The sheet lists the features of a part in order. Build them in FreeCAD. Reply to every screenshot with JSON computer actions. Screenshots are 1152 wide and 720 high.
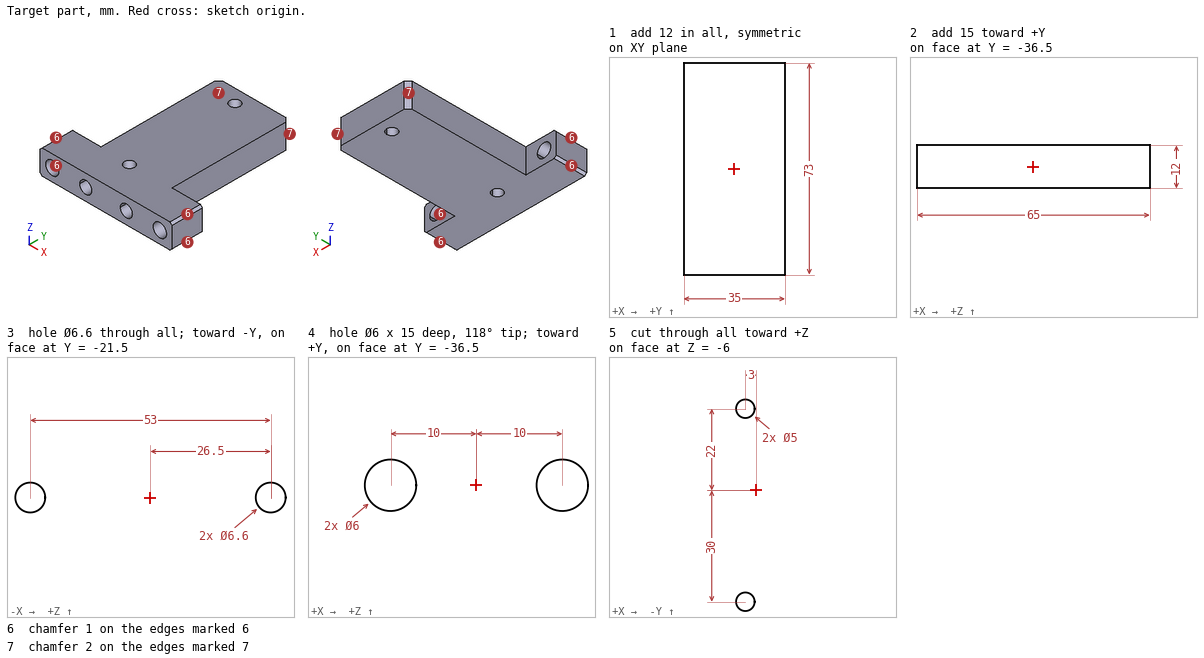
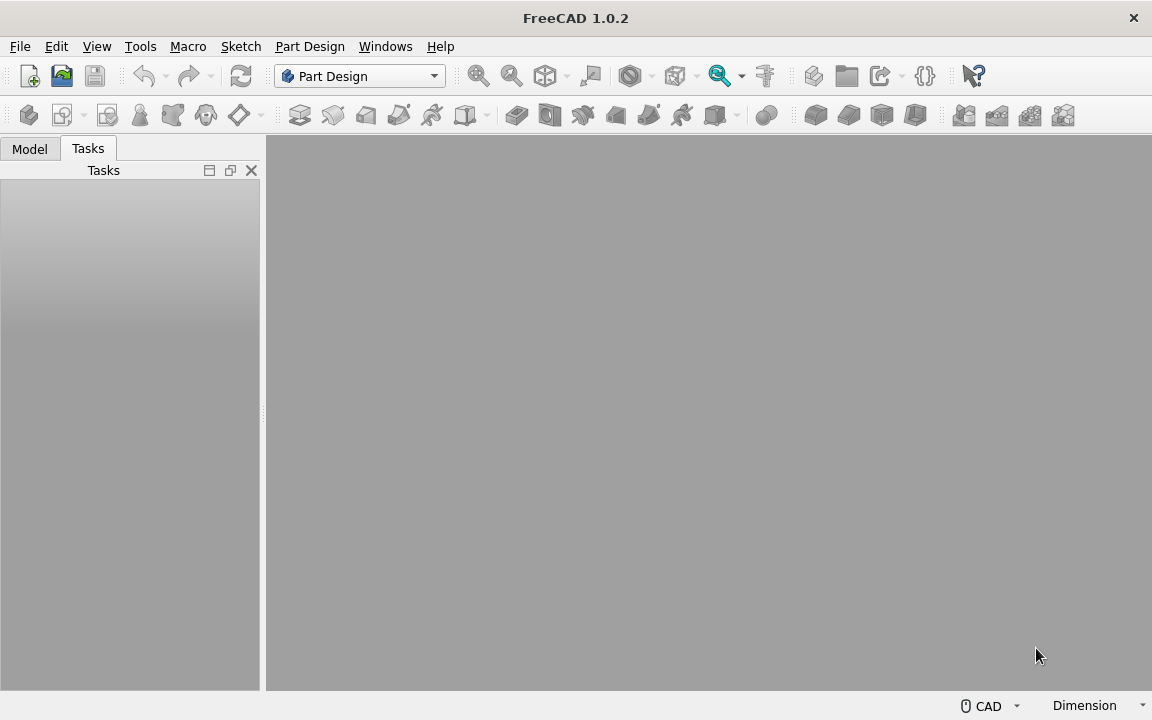
{"action": "left_click", "coordinate": [29, 76]}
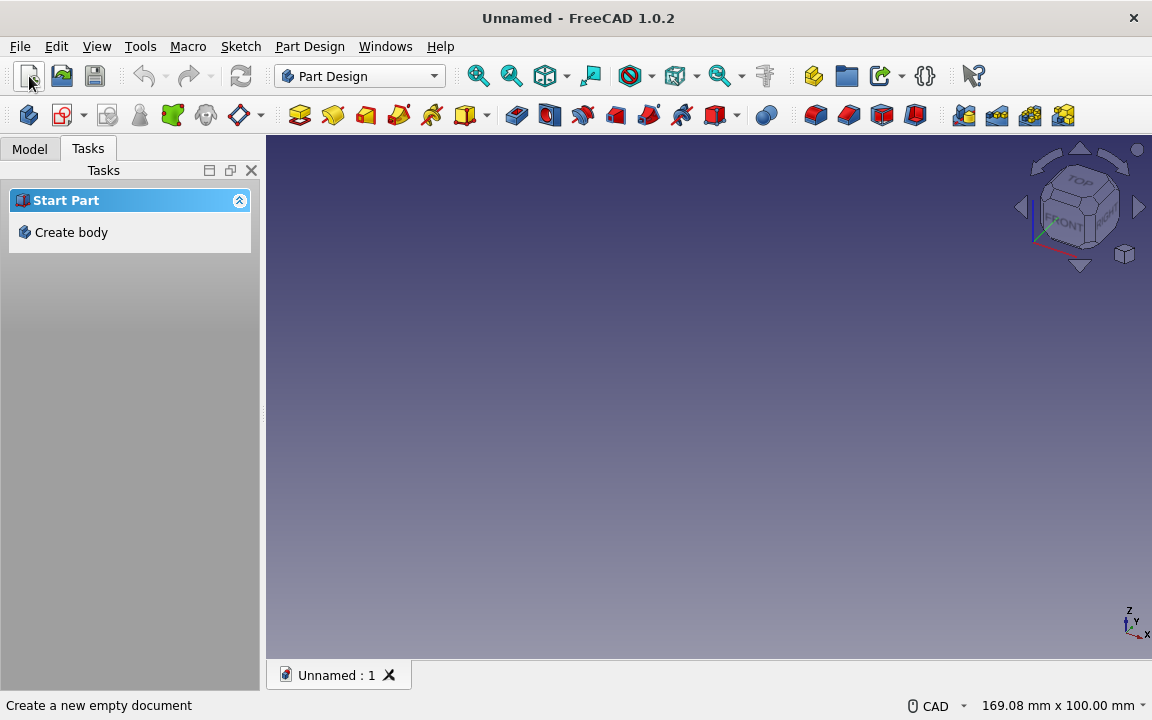
{"action": "left_click", "coordinate": [62, 116]}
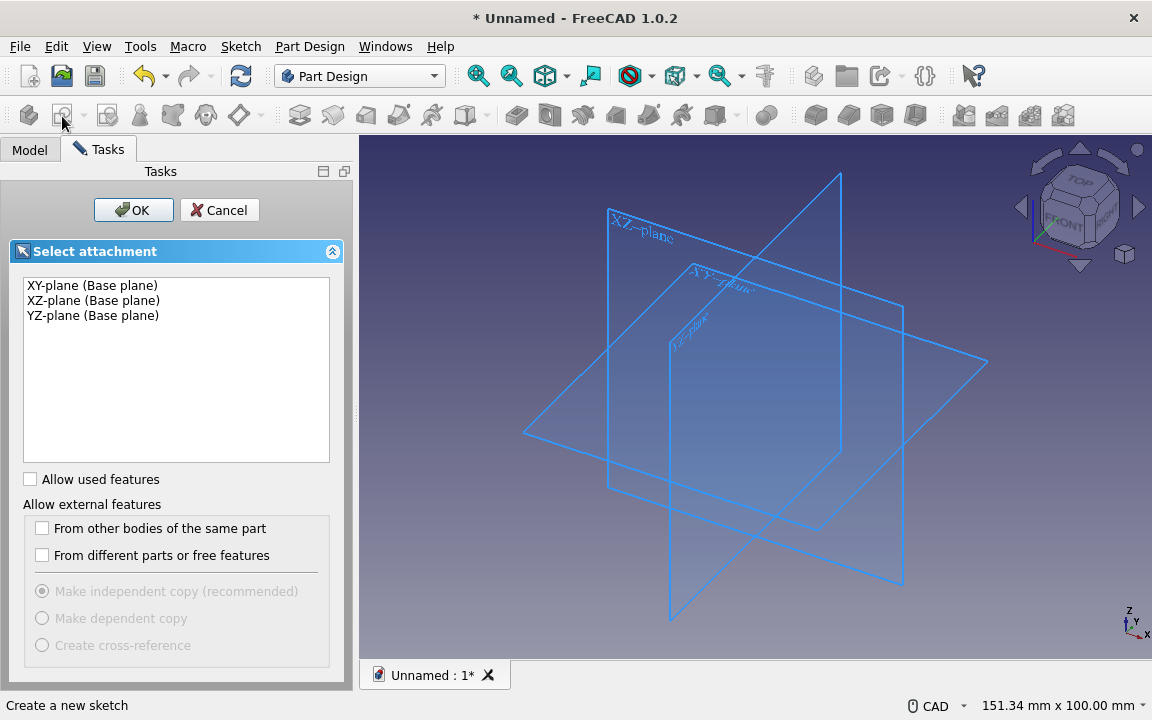
{"action": "left_click", "coordinate": [84, 286]}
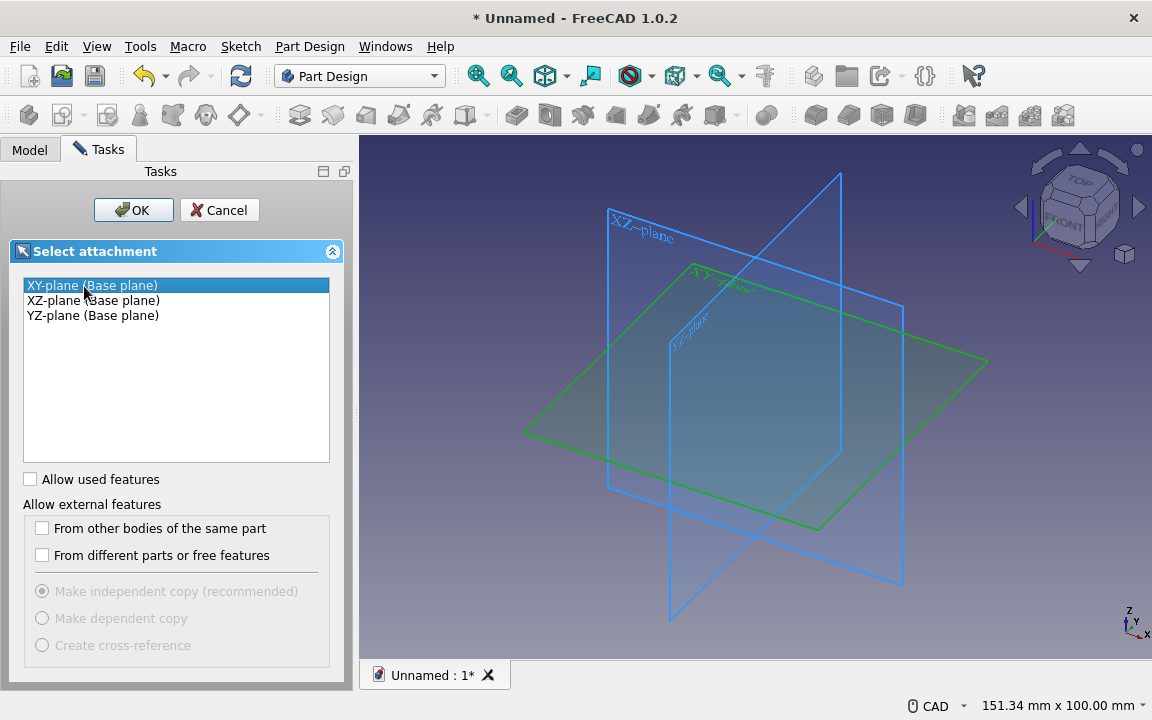
{"action": "left_click", "coordinate": [134, 210]}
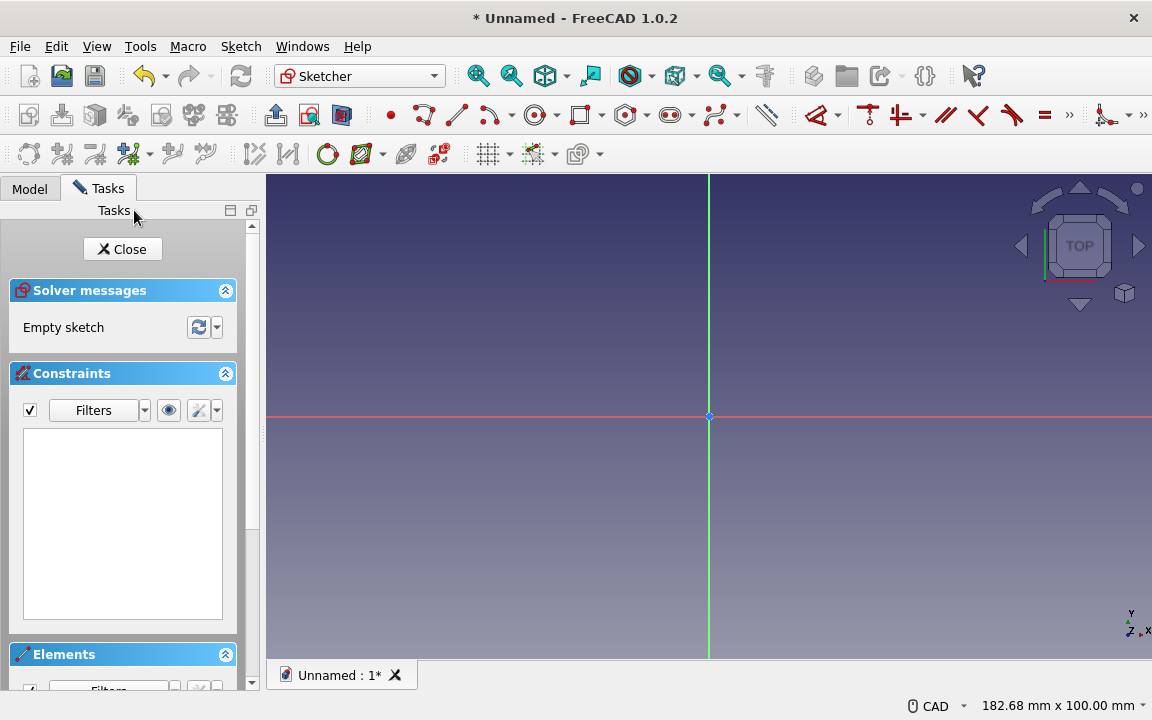
{"action": "key", "text": "g v"}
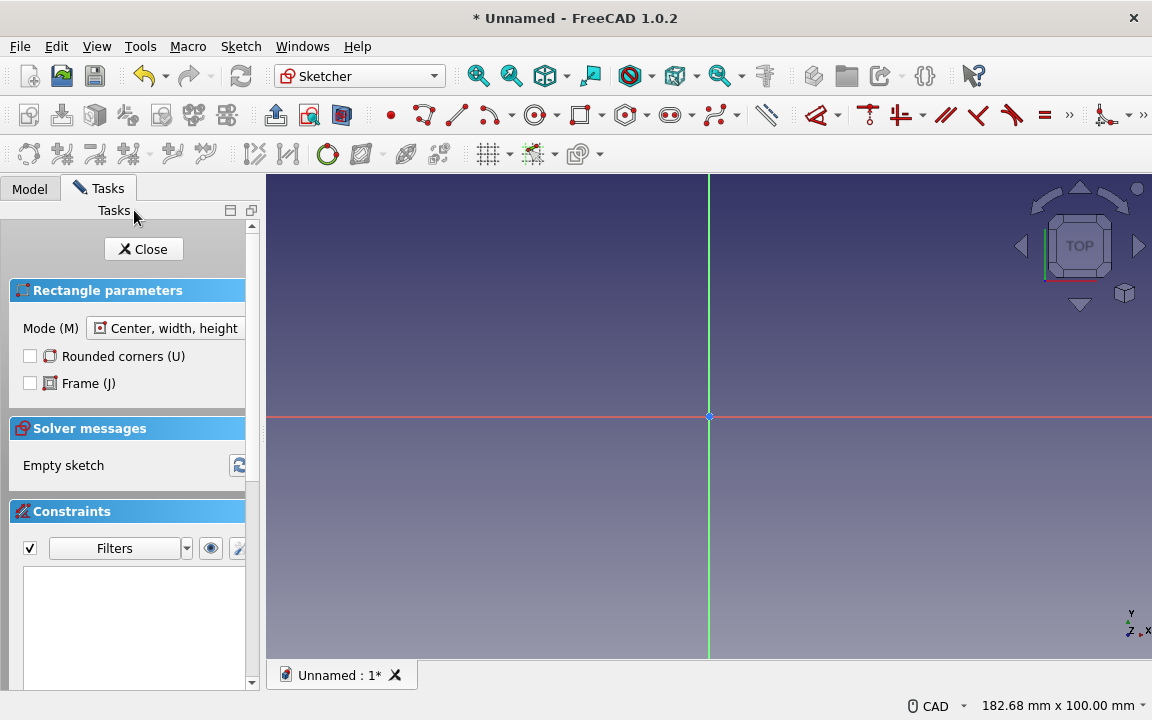
{"action": "left_click", "coordinate": [709, 416]}
{"action": "mouse_move", "coordinate": [794, 239]}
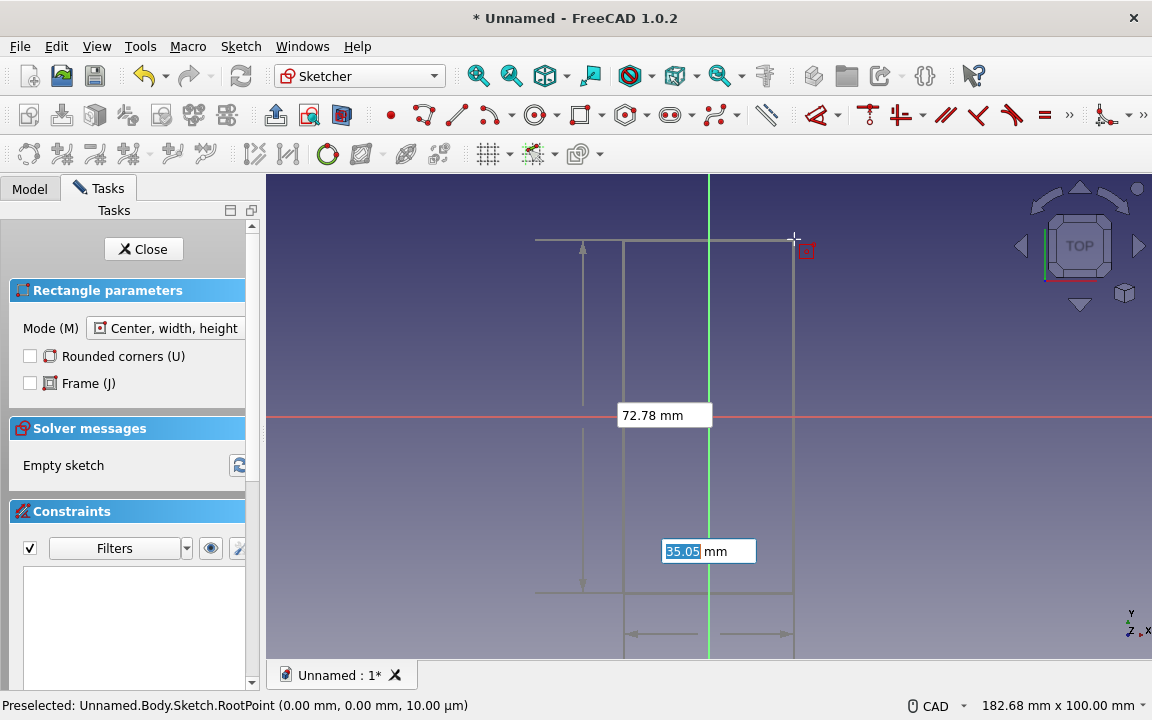
{"action": "type", "text": "35"}
{"action": "key", "text": "Tab"}
{"action": "type", "text": "73"}
{"action": "key", "text": "Return"}
{"action": "key", "text": "Escape"}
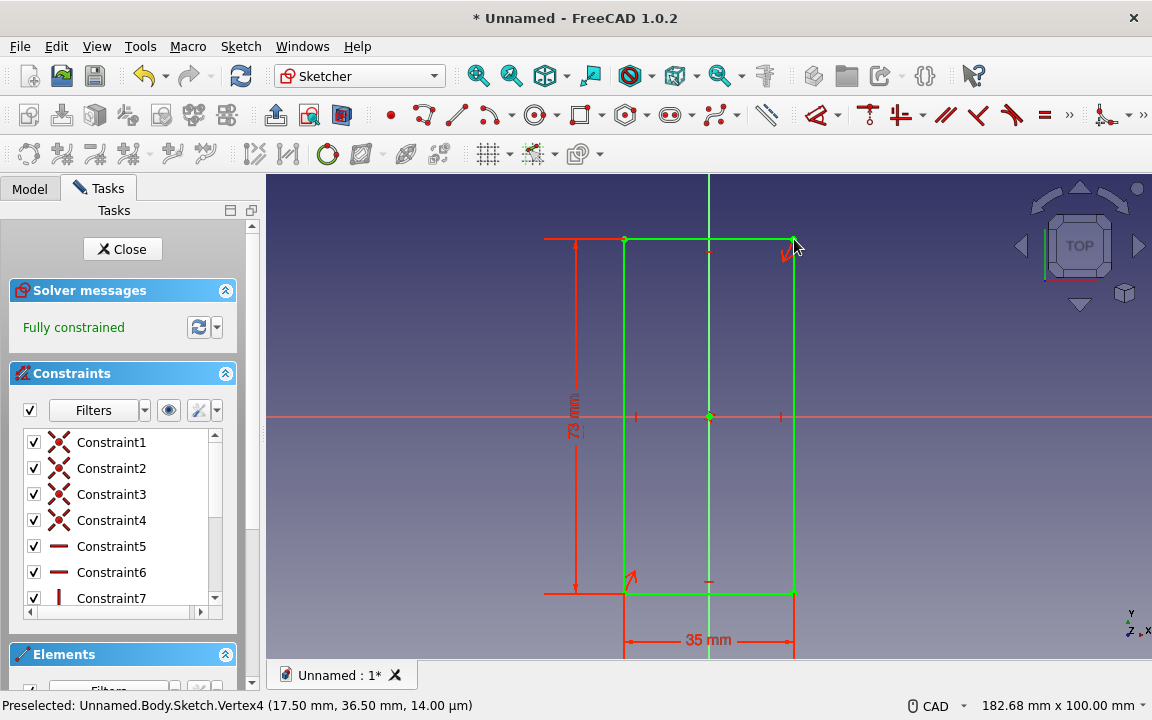
{"action": "left_click", "coordinate": [123, 249]}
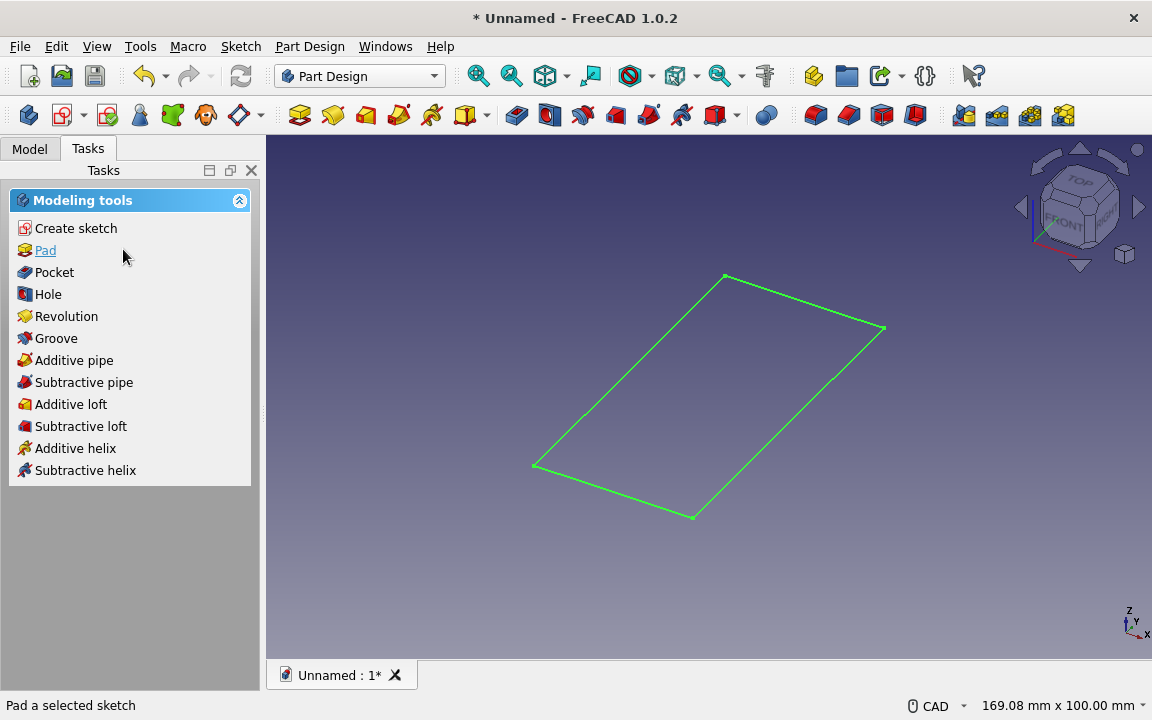
{"action": "left_click", "coordinate": [300, 116]}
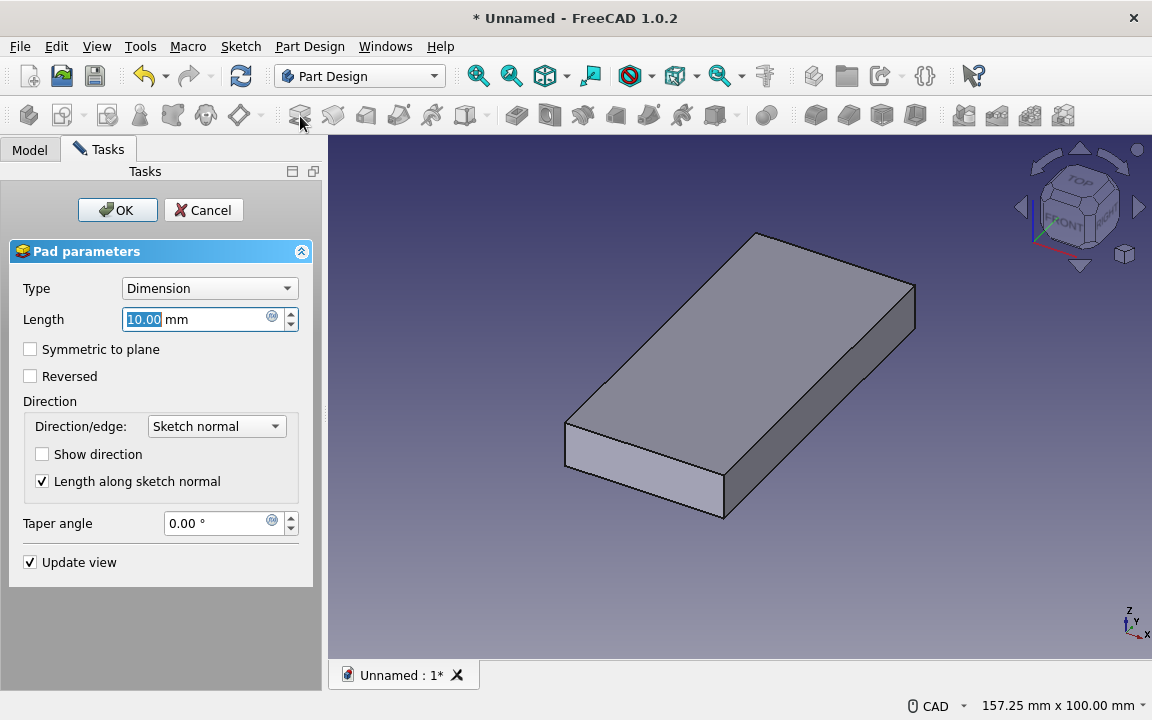
{"action": "type", "text": "12"}
{"action": "key", "text": "Tab"}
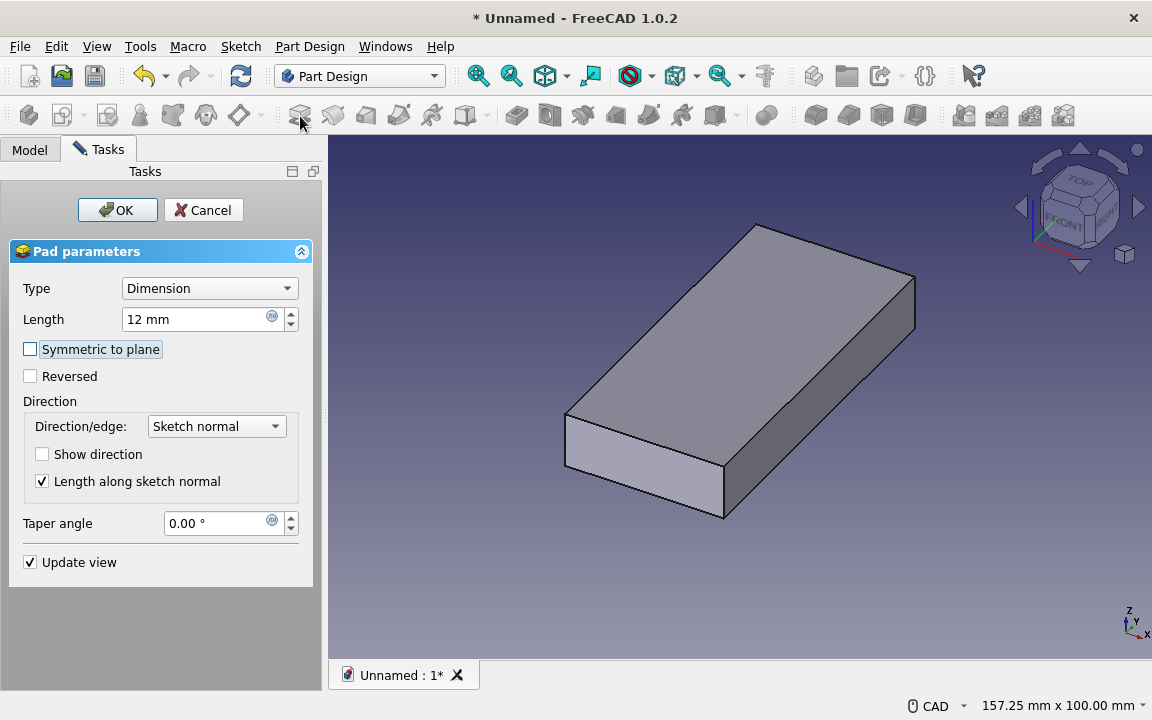
{"action": "left_click", "coordinate": [31, 349]}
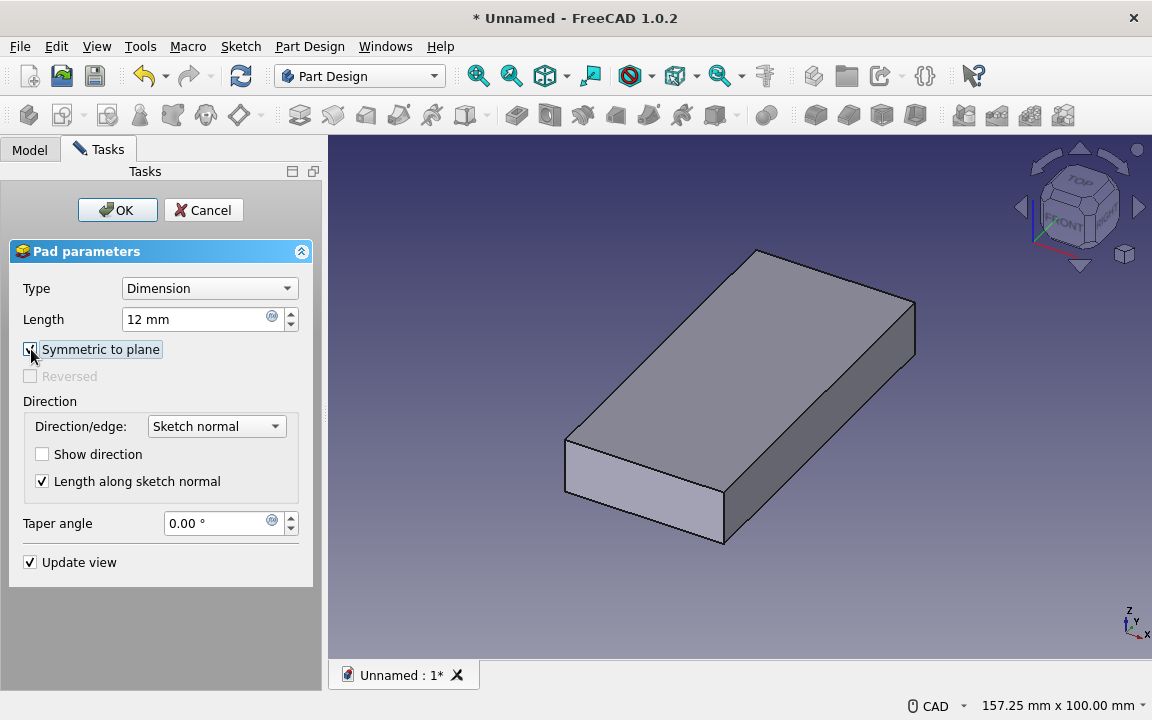
{"action": "left_click", "coordinate": [118, 210]}